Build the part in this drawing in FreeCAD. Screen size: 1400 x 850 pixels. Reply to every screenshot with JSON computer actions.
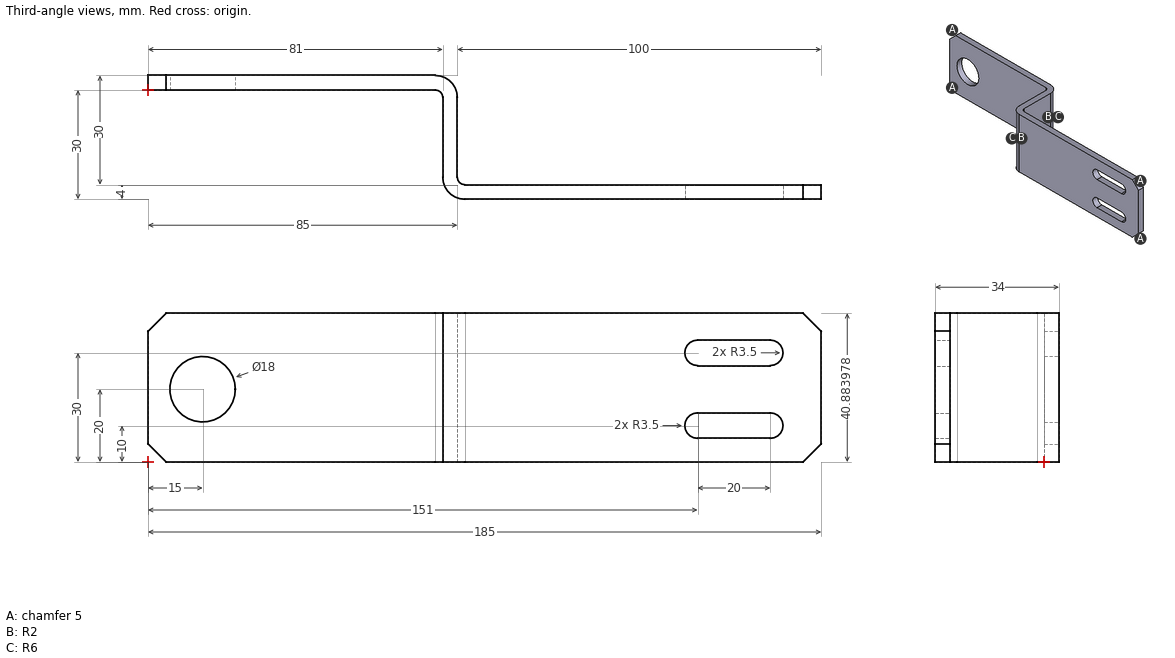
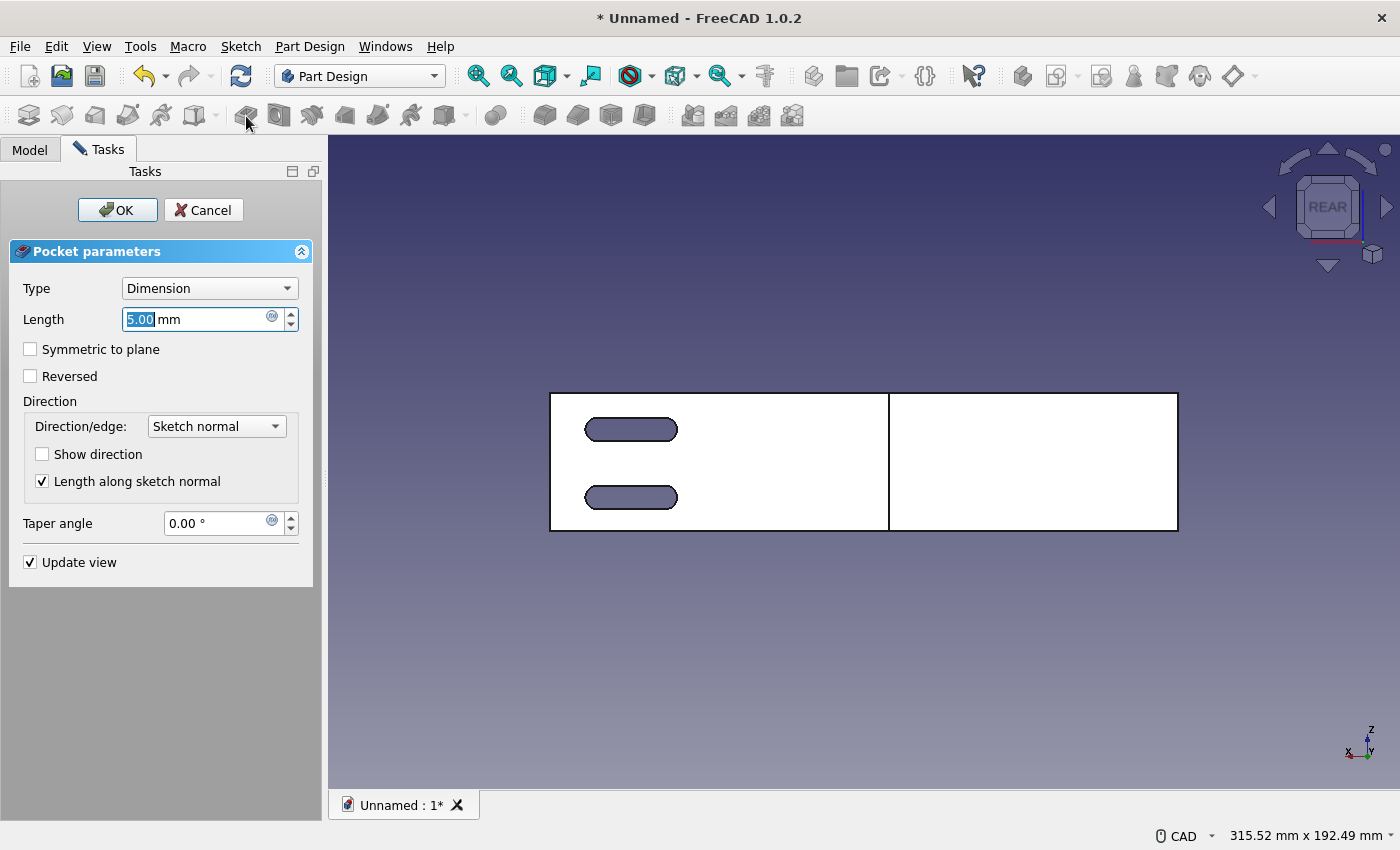
{"action": "left_click", "coordinate": [210, 288]}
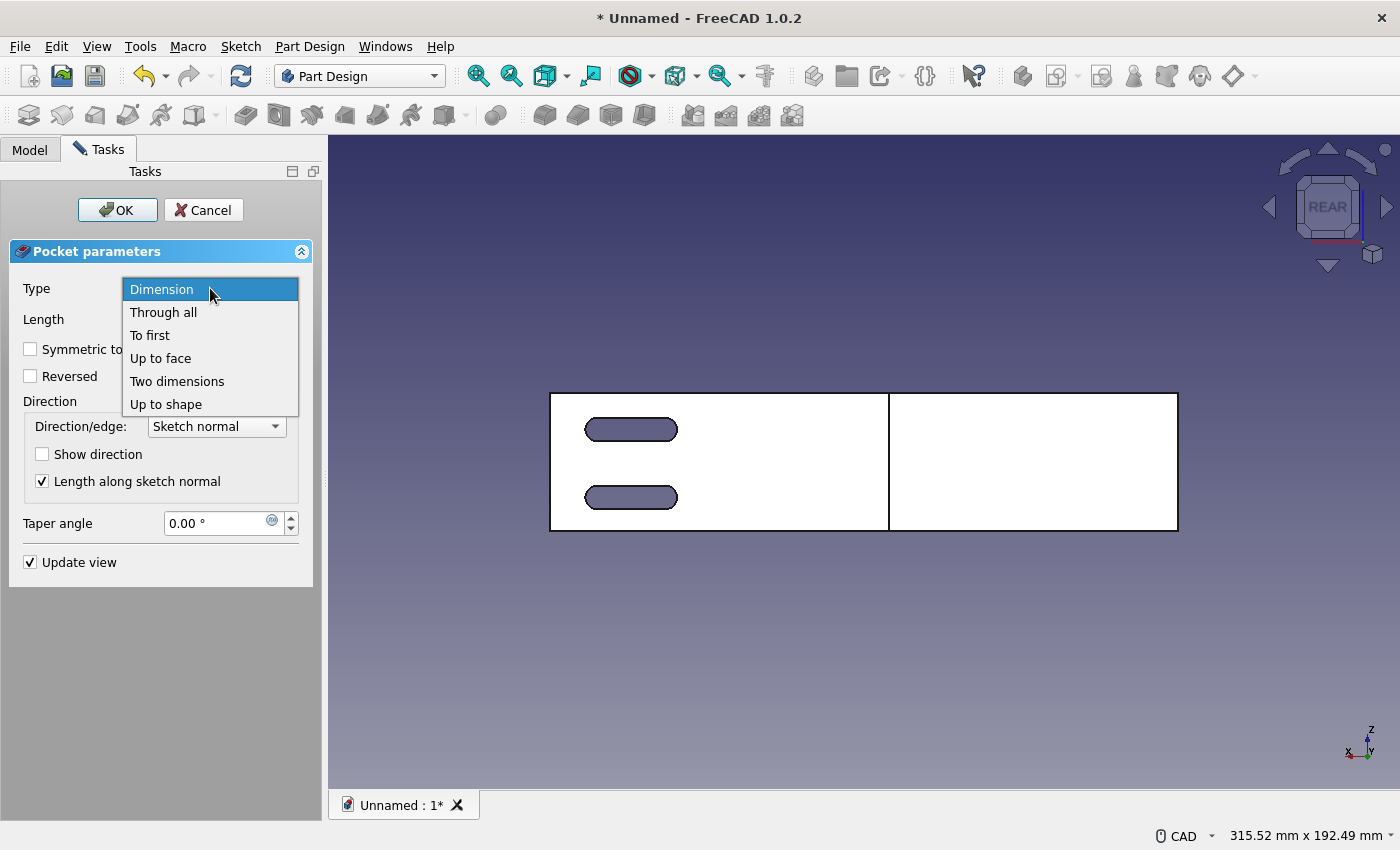
{"action": "left_click", "coordinate": [208, 312]}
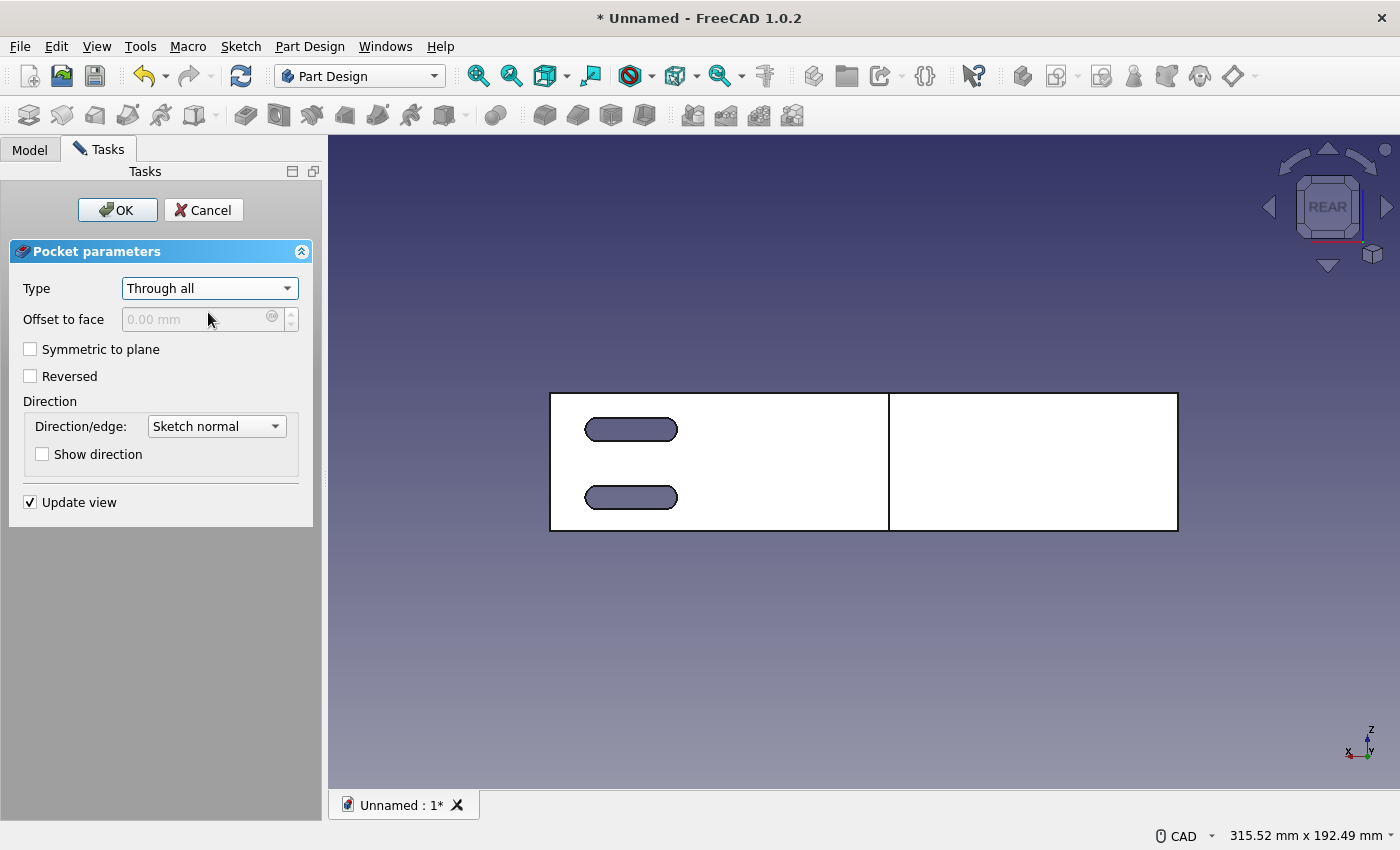
{"action": "left_click", "coordinate": [118, 210]}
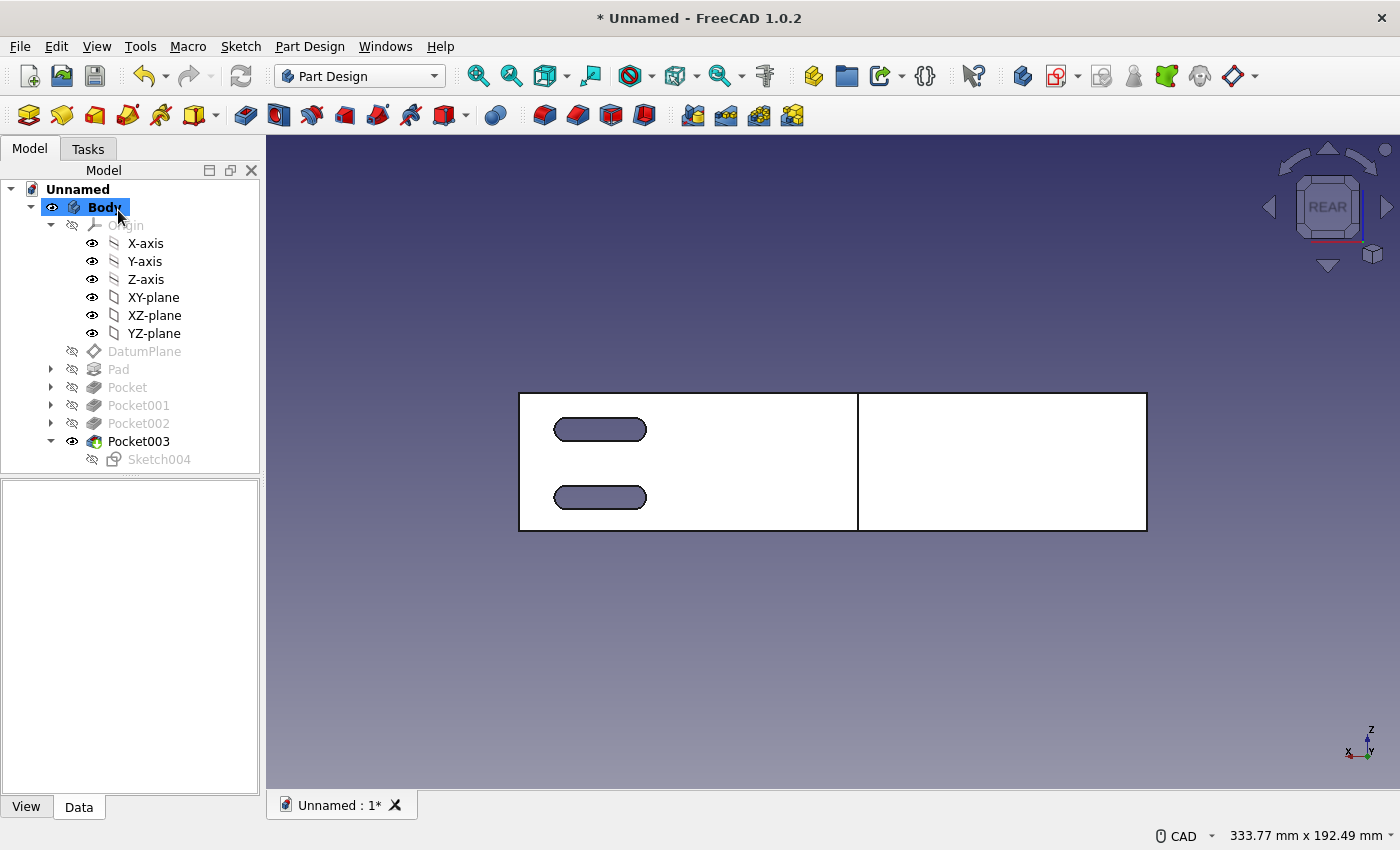
{"action": "key", "text": "0"}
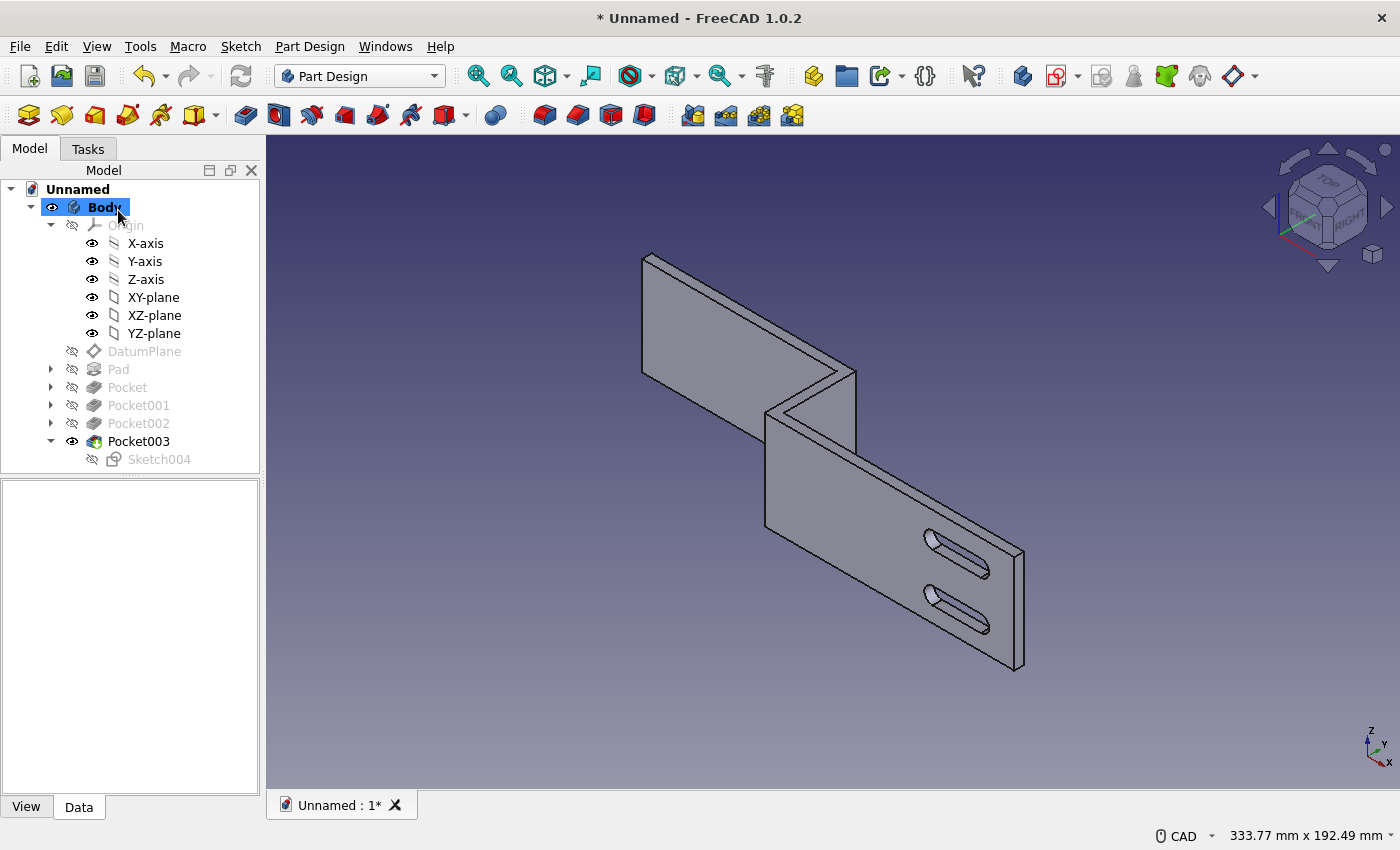
{"action": "left_click", "coordinate": [767, 387]}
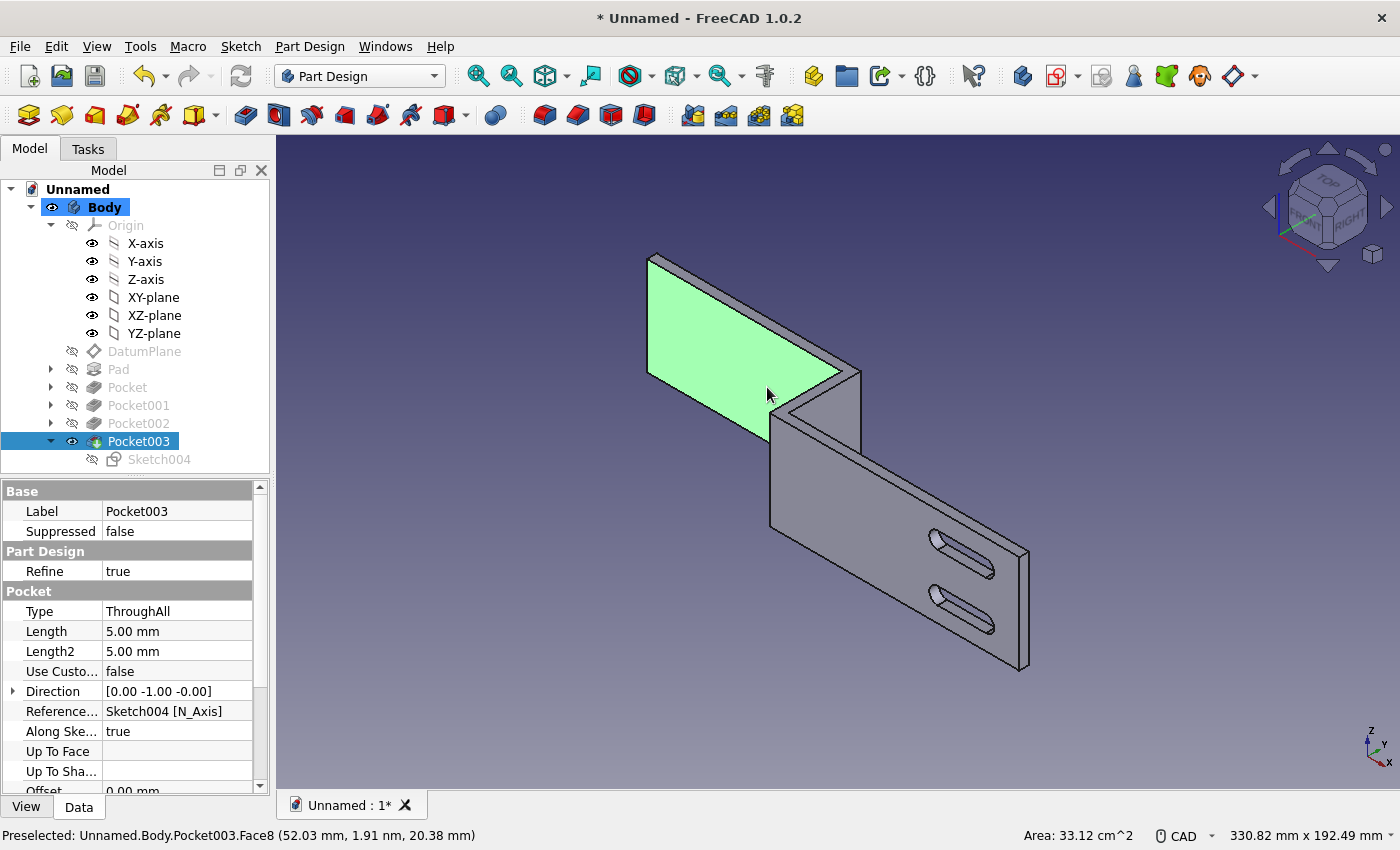
{"action": "left_click", "coordinate": [1056, 76]}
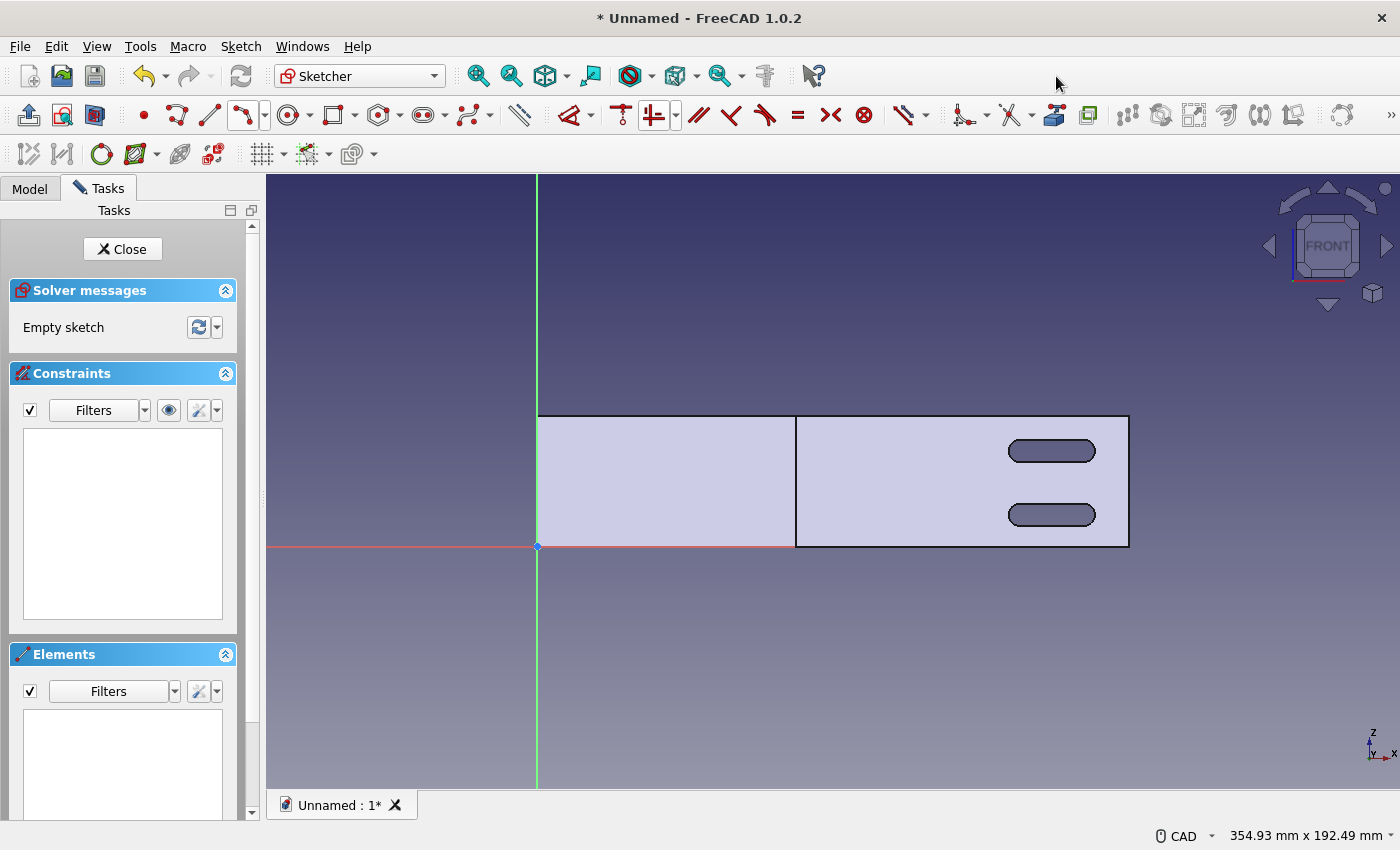
{"action": "scroll", "coordinate": [514, 507], "scroll_direction": "up", "scroll_amount": 7}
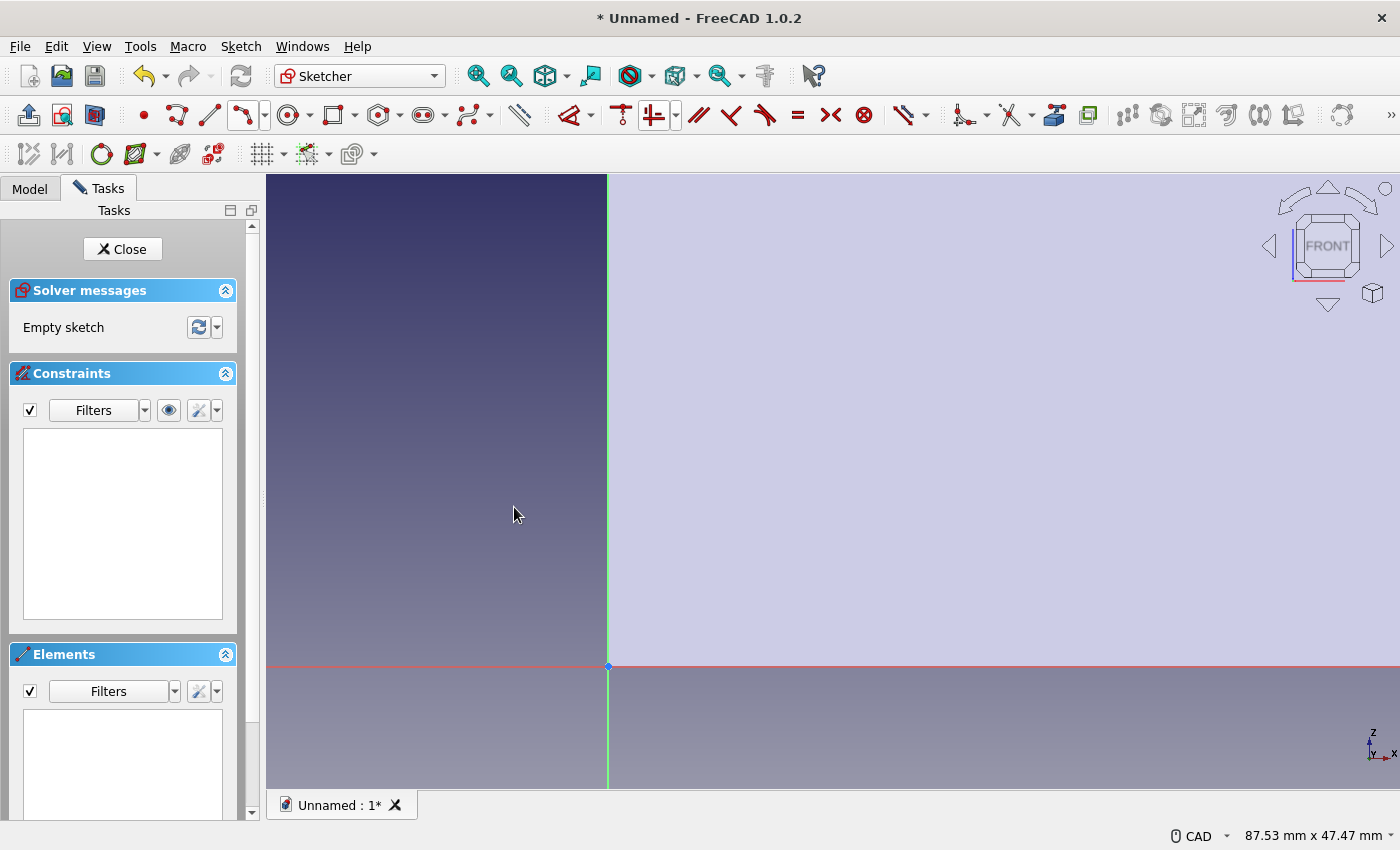
{"action": "left_click", "coordinate": [288, 116]}